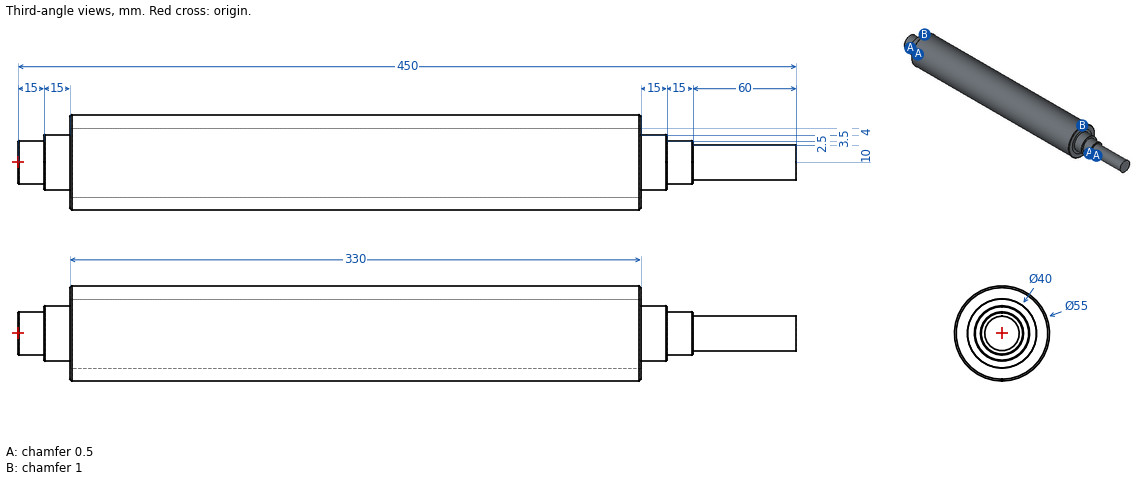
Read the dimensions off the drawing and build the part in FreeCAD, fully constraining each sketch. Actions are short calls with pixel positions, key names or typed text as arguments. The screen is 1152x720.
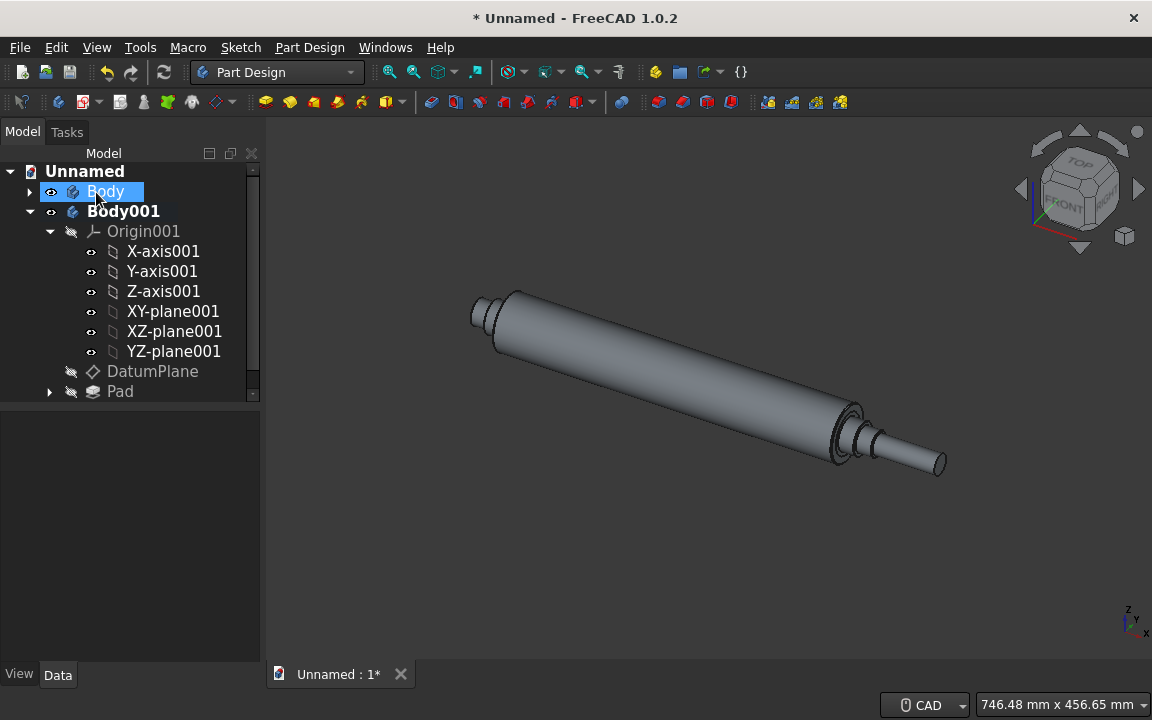
key(0)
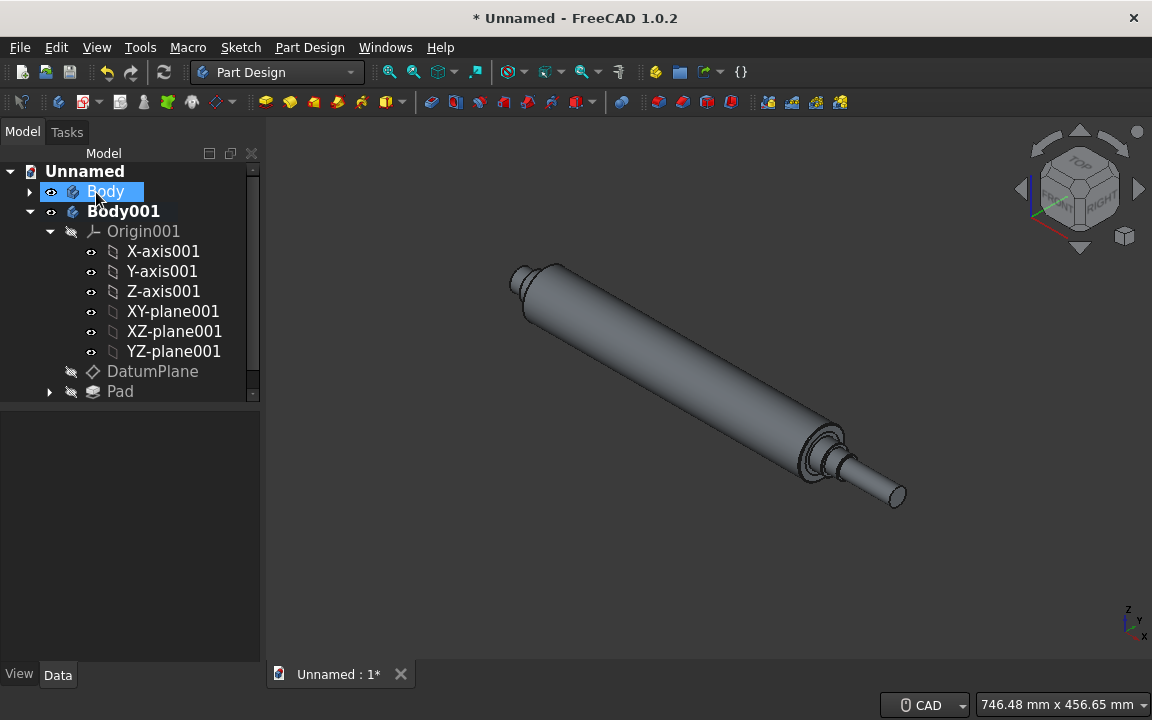
click(390, 72)